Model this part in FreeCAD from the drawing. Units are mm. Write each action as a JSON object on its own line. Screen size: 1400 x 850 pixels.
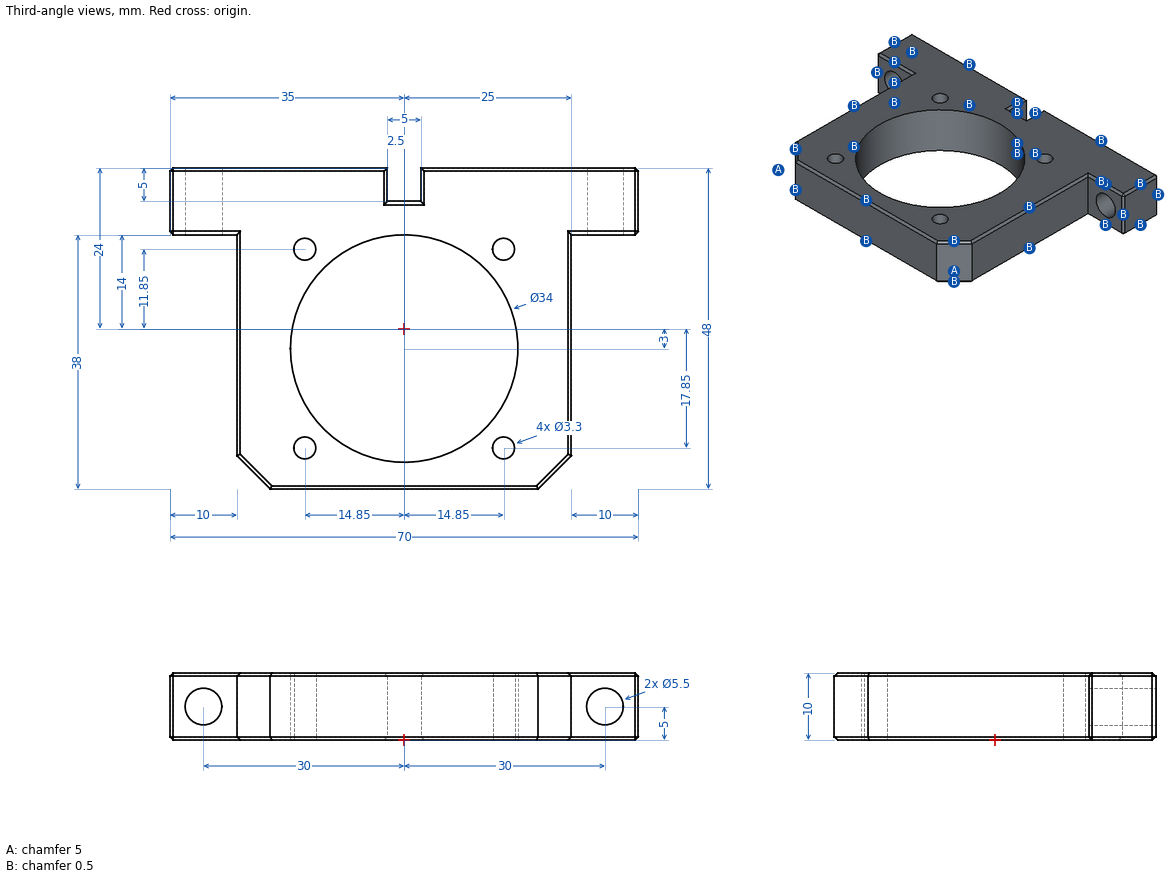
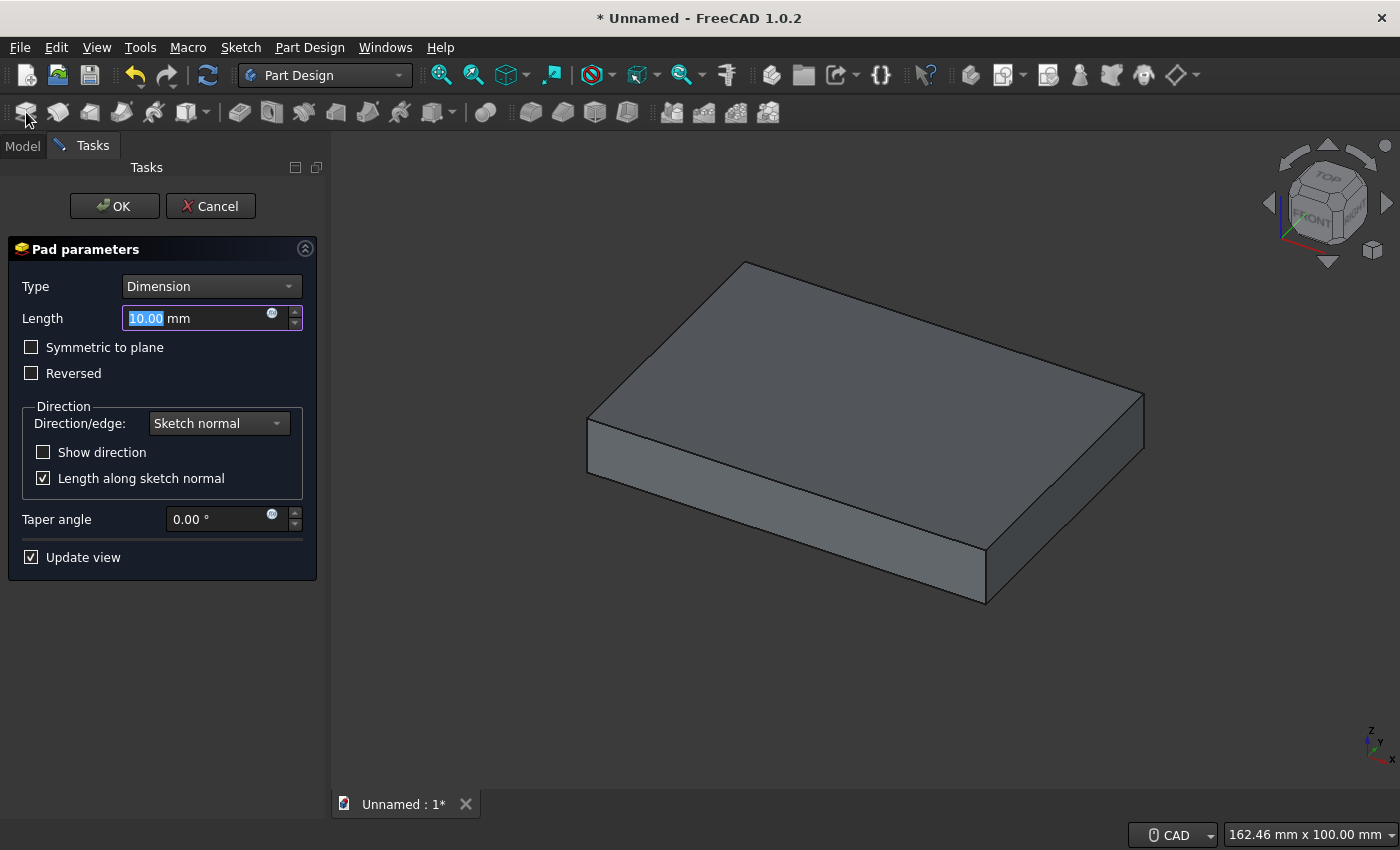
{"action": "type", "text": "10"}
{"action": "key", "text": "Tab"}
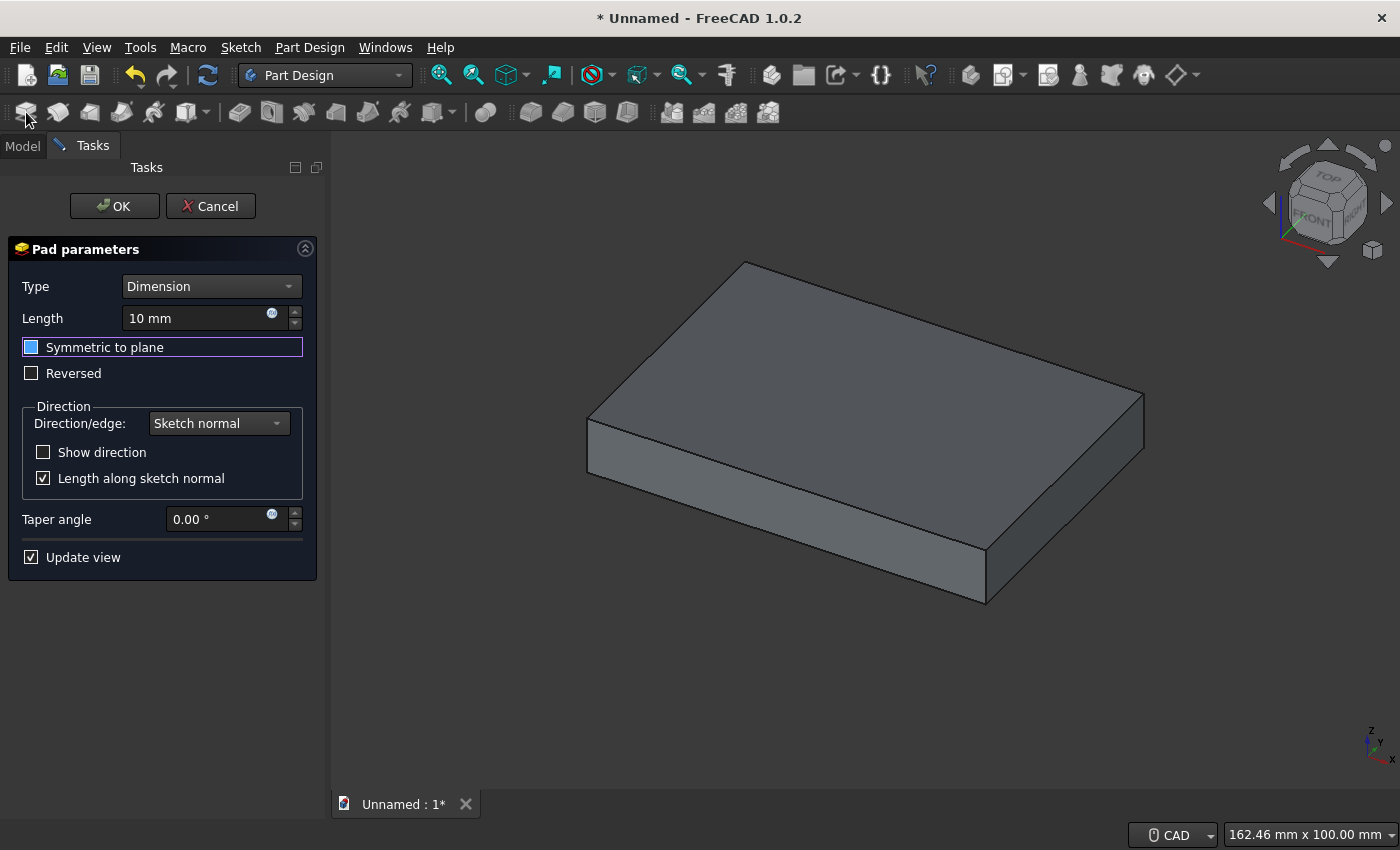
{"action": "left_click", "coordinate": [115, 206]}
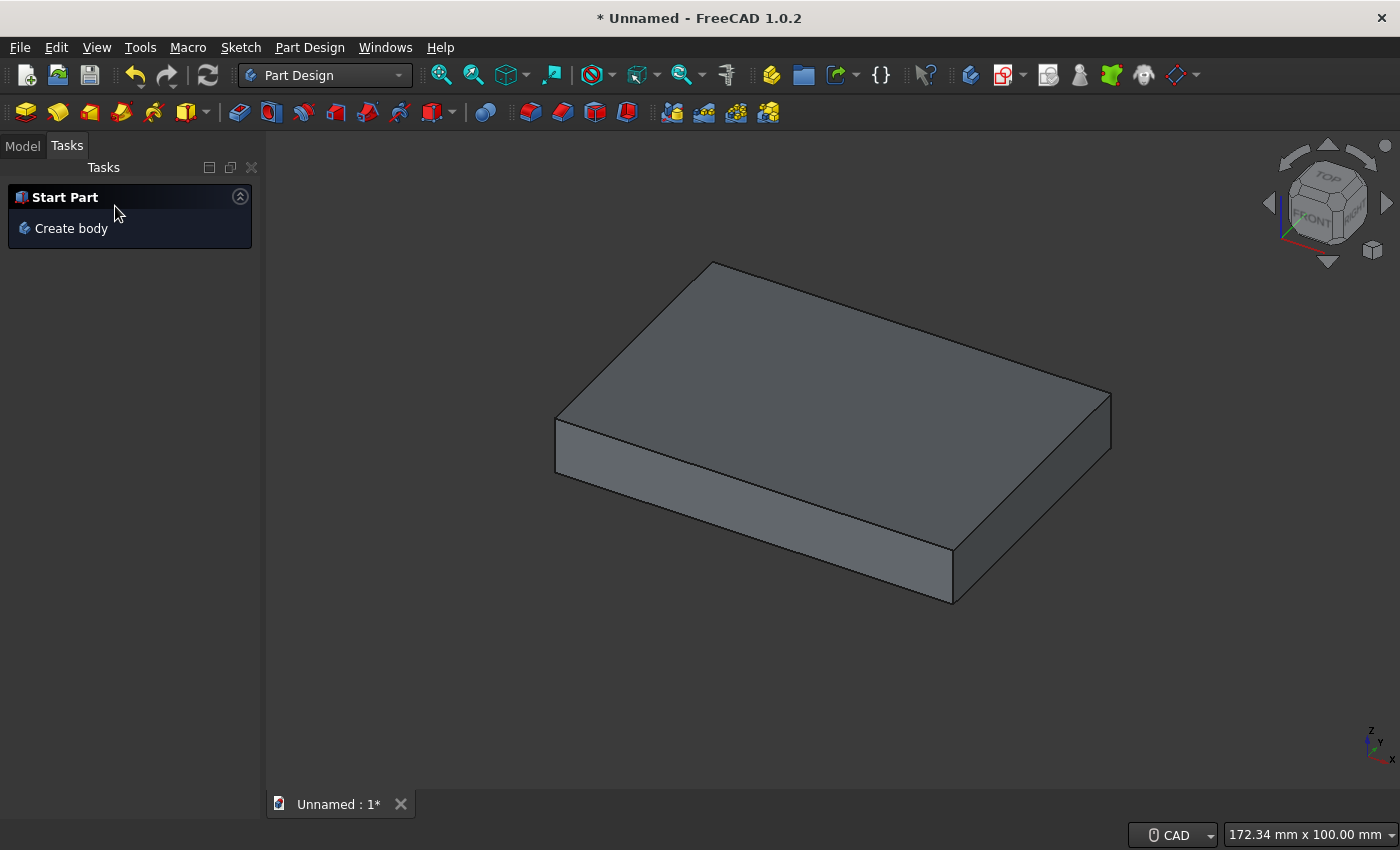
{"action": "left_click", "coordinate": [890, 424]}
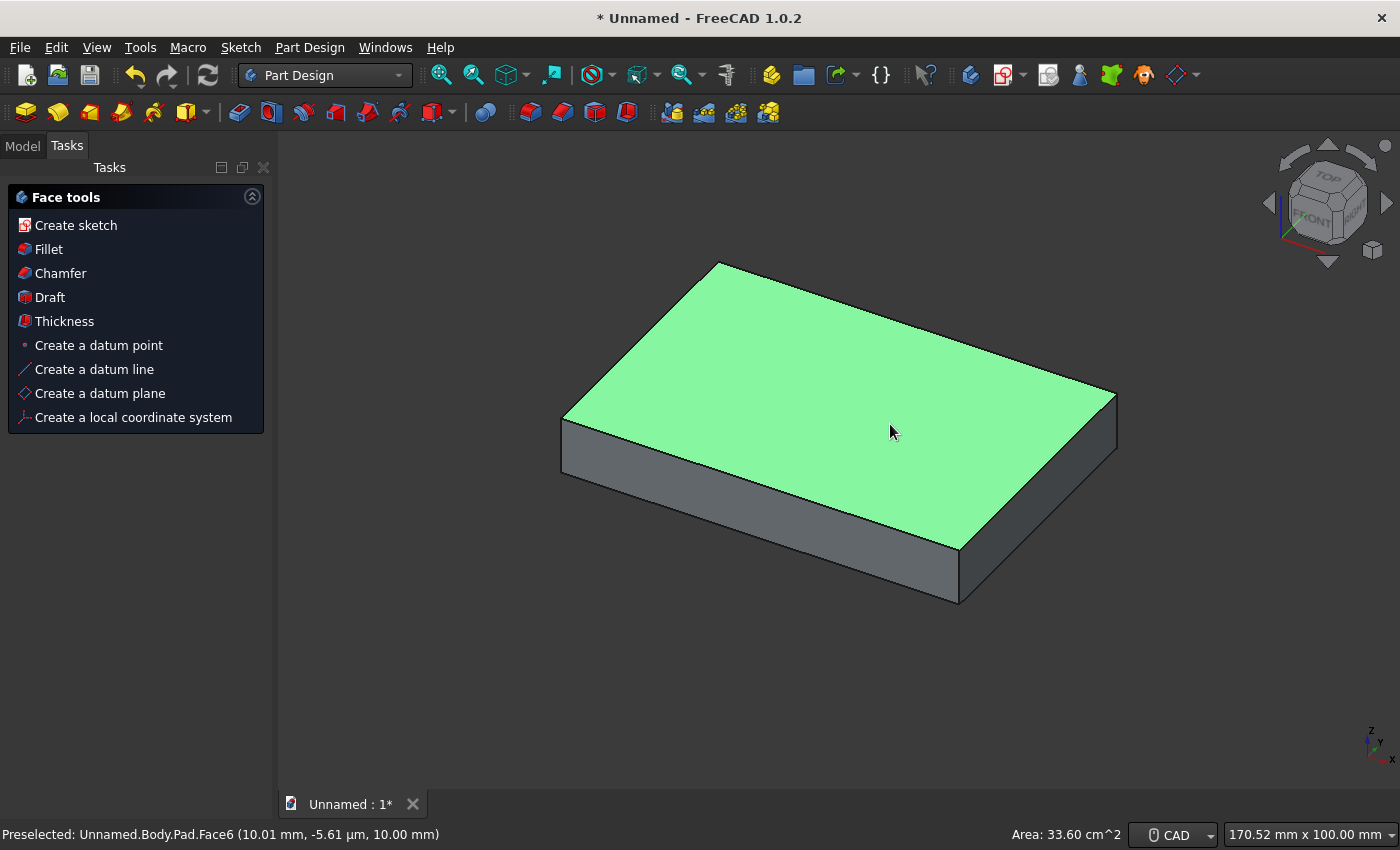
{"action": "left_click", "coordinate": [1004, 76]}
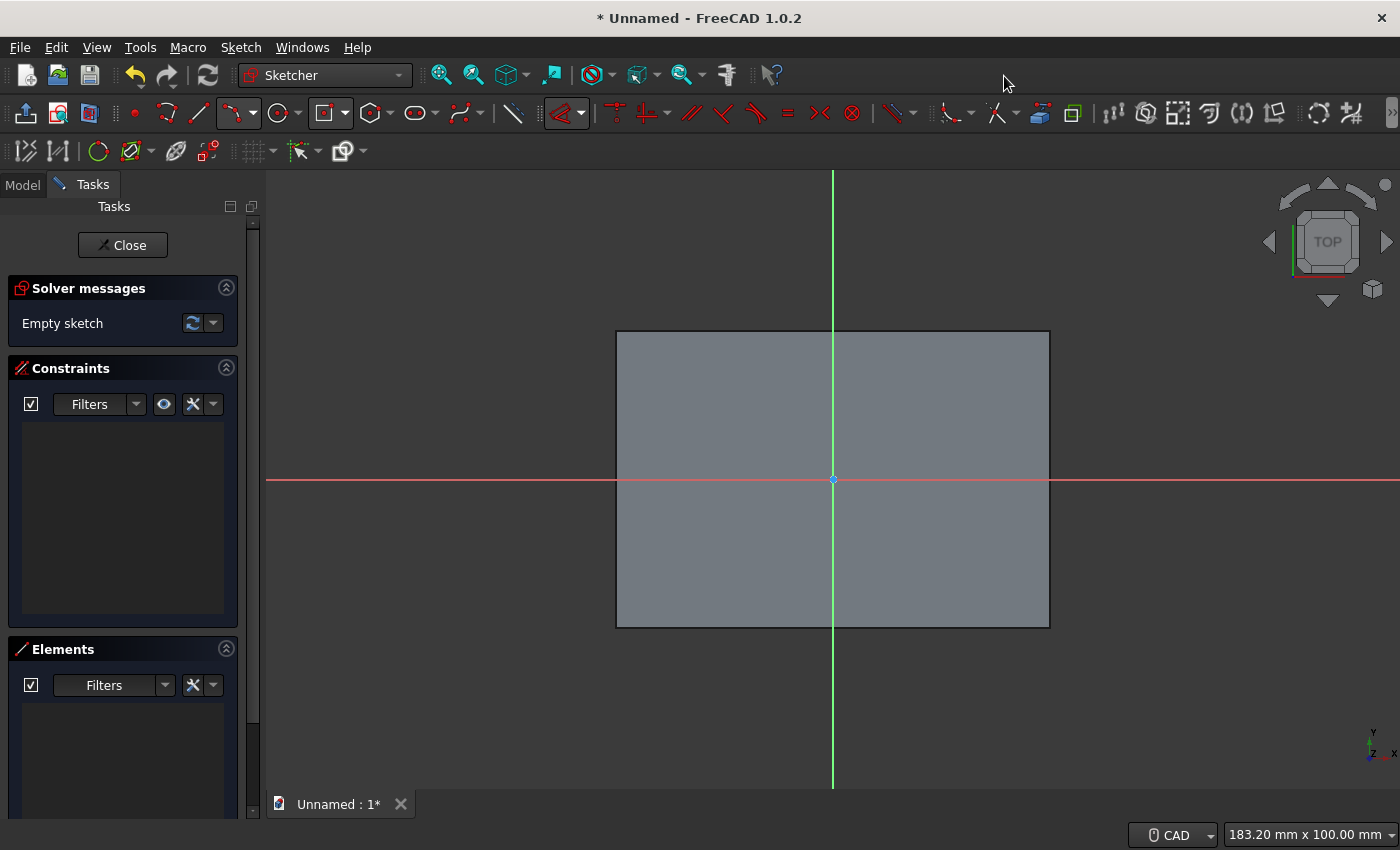
{"action": "scroll", "coordinate": [972, 573], "scroll_direction": "up", "scroll_amount": 2}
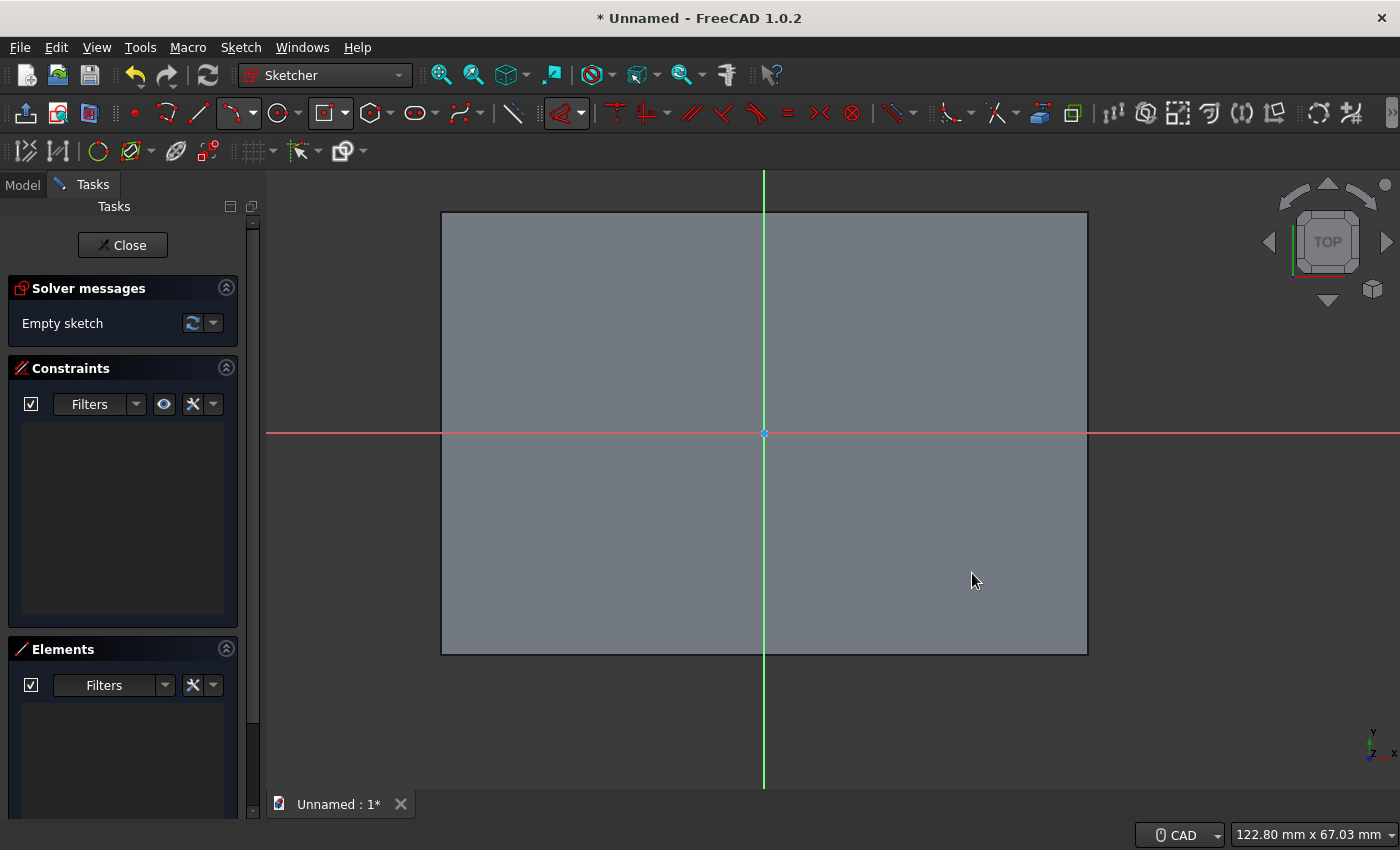
{"action": "left_click", "coordinate": [348, 114]}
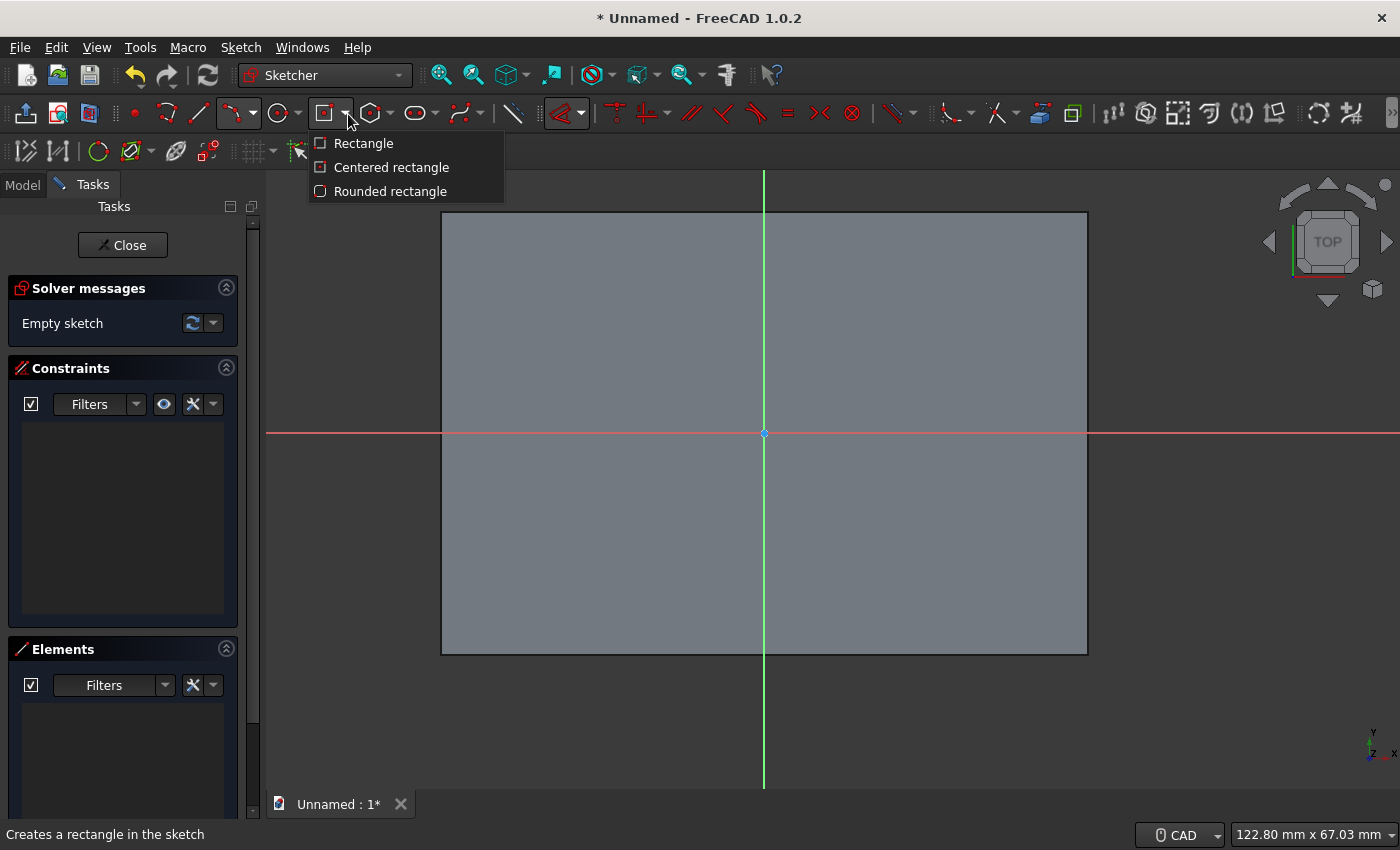
{"action": "left_click", "coordinate": [406, 143]}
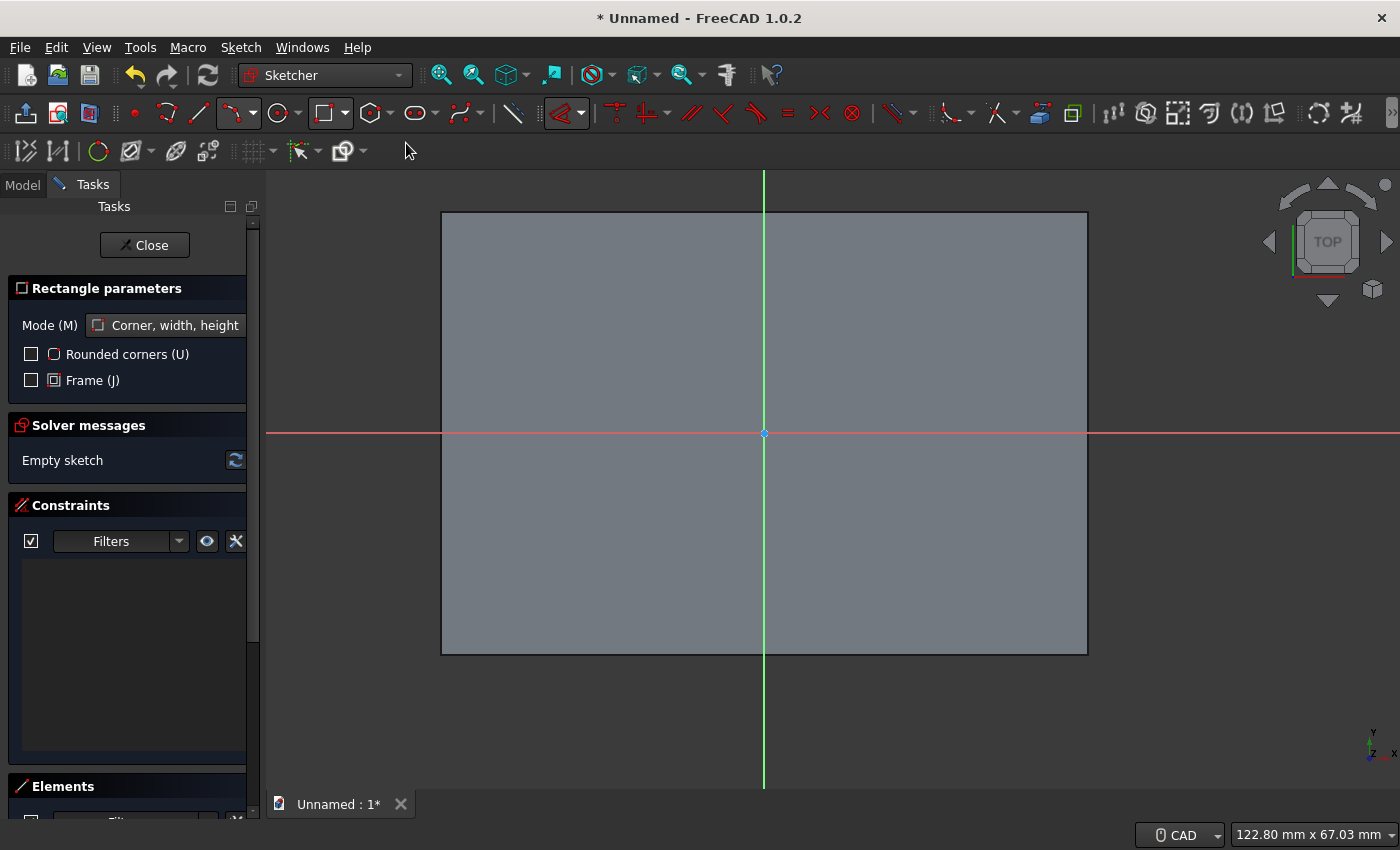
{"action": "left_click", "coordinate": [441, 304]}
{"action": "left_click", "coordinate": [533, 655]}